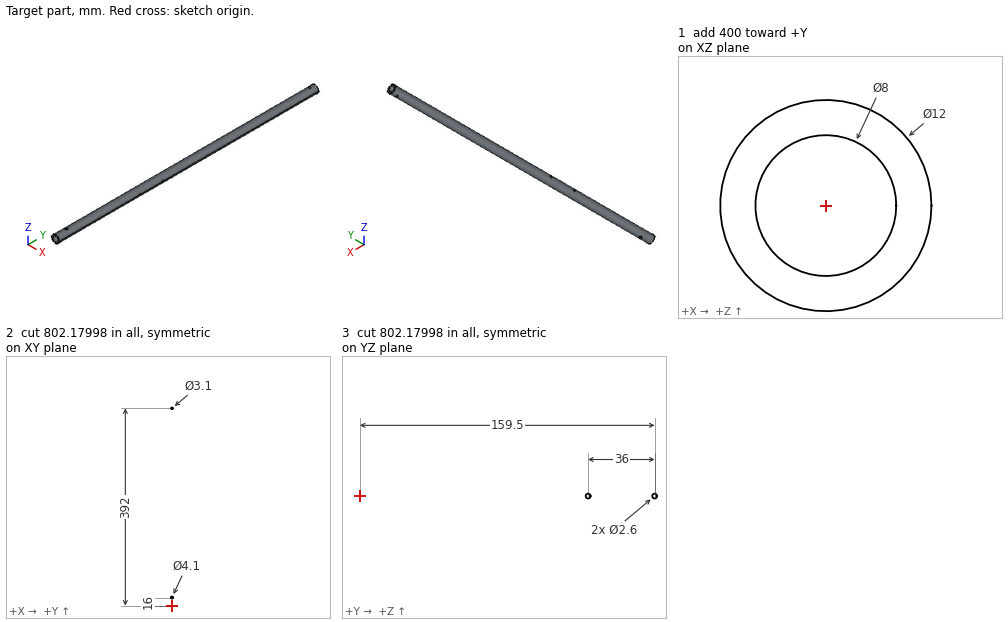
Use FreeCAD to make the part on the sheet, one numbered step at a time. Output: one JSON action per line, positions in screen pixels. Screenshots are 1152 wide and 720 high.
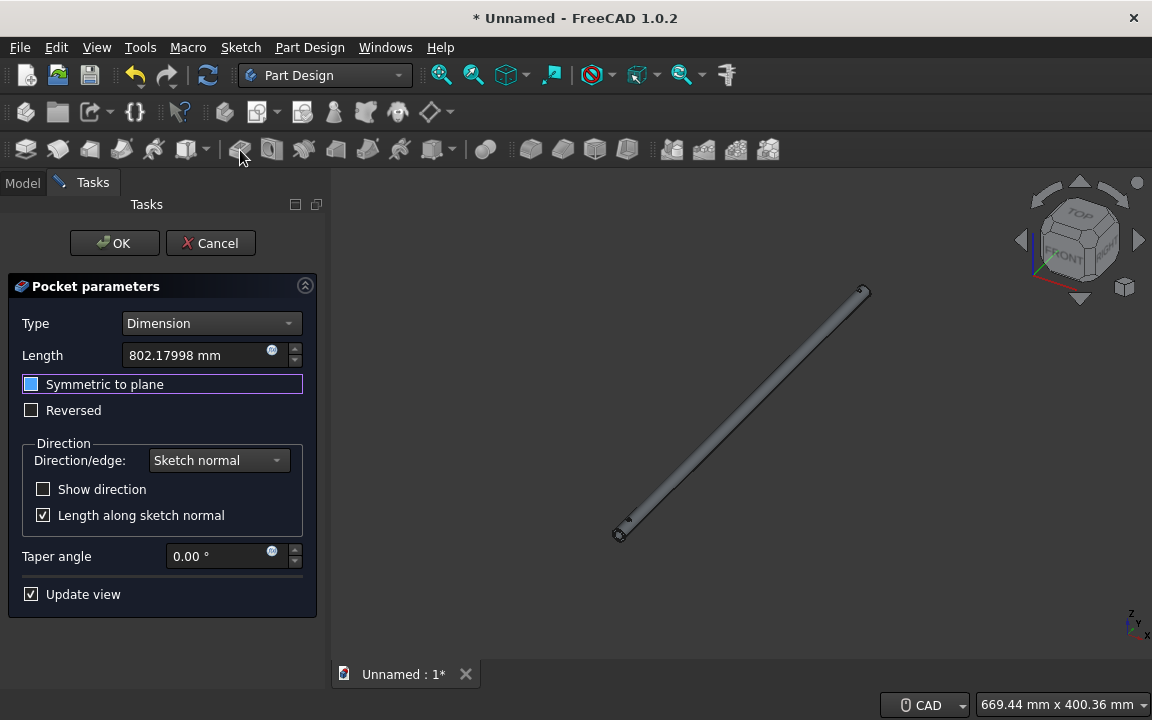
{"action": "left_click", "coordinate": [30, 384]}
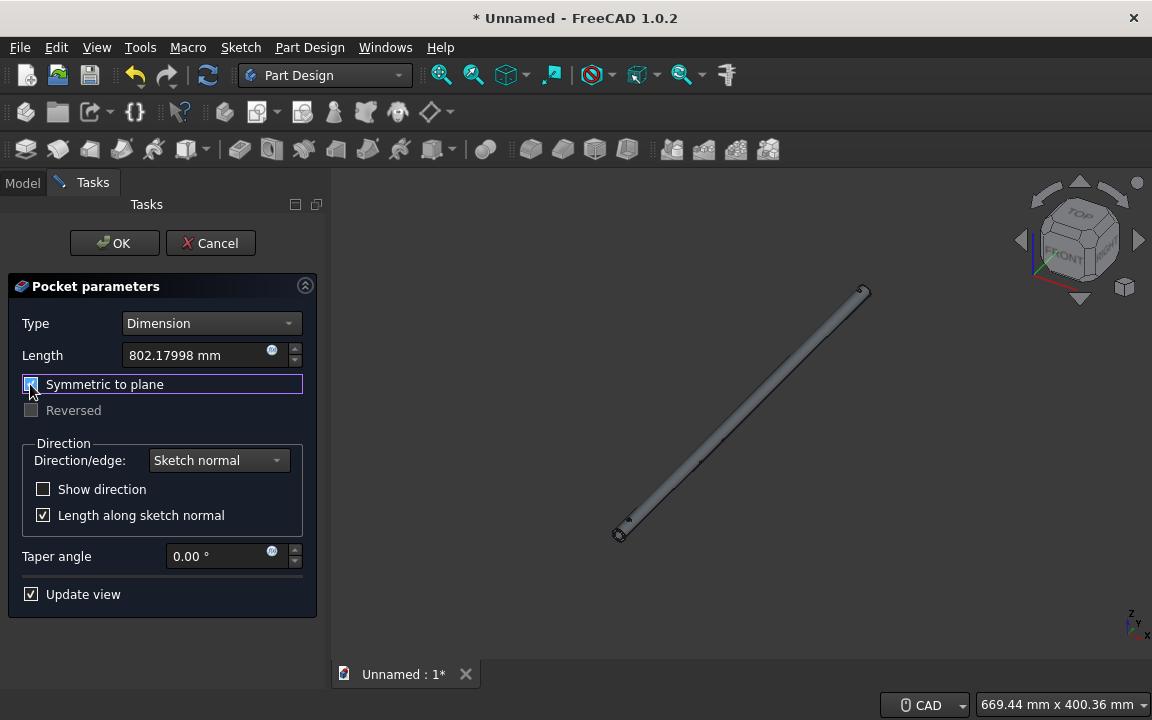
{"action": "left_click", "coordinate": [115, 243]}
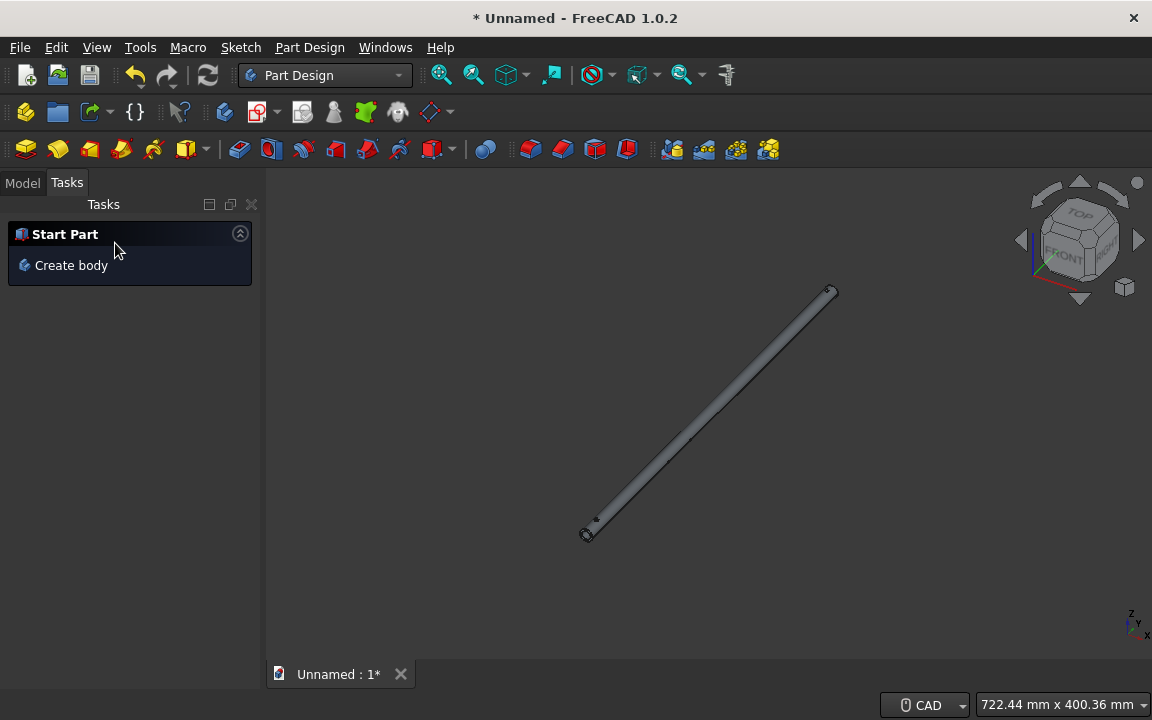
{"action": "key", "text": "0"}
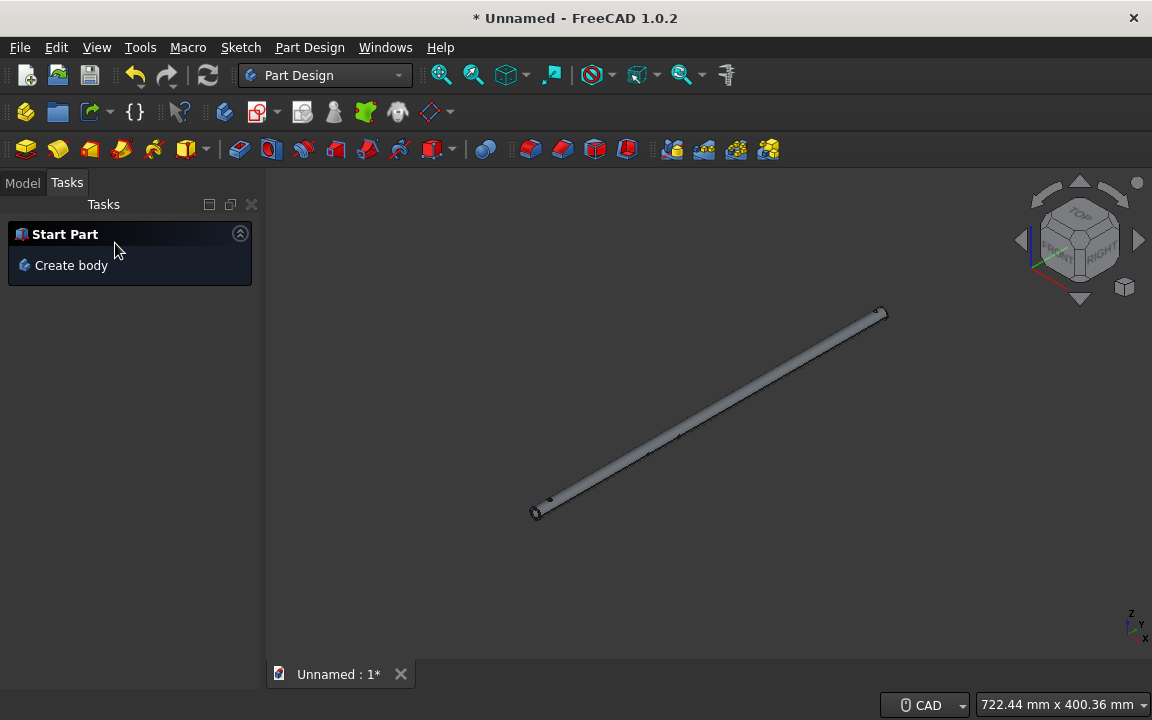
{"action": "left_click", "coordinate": [442, 76]}